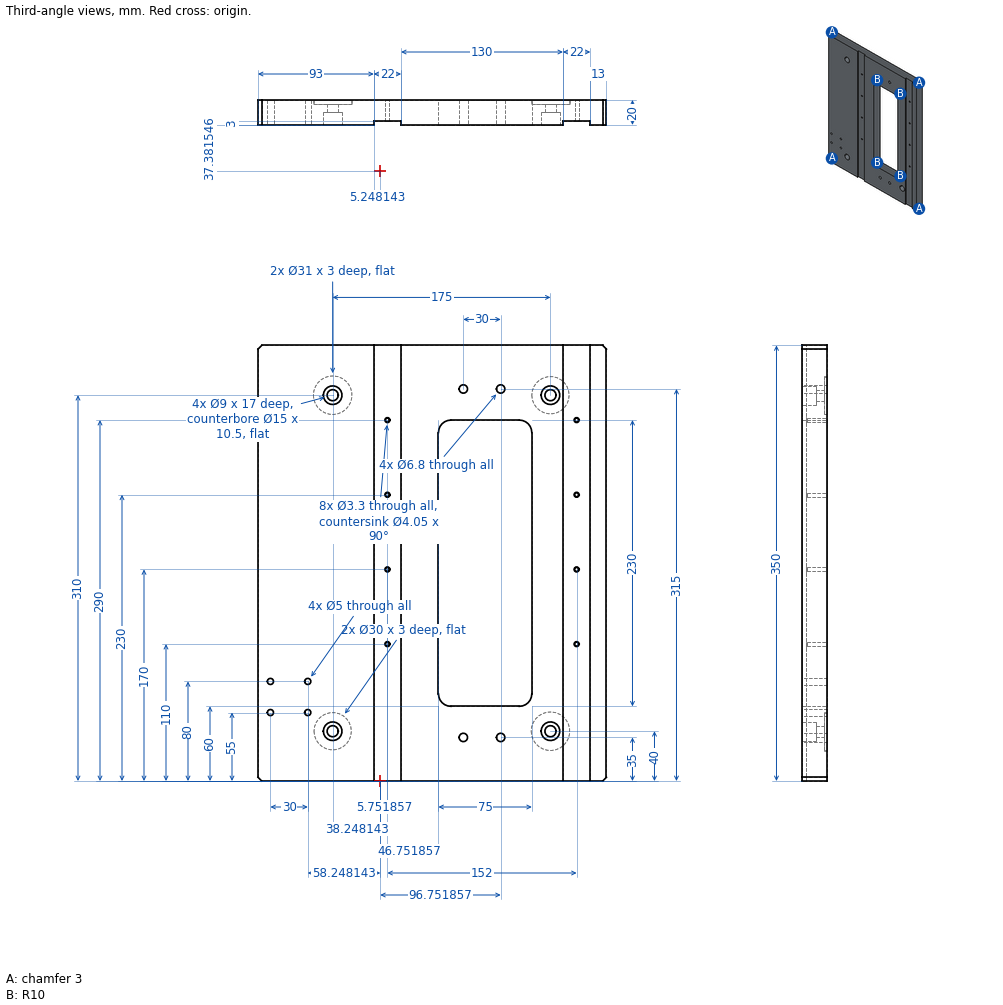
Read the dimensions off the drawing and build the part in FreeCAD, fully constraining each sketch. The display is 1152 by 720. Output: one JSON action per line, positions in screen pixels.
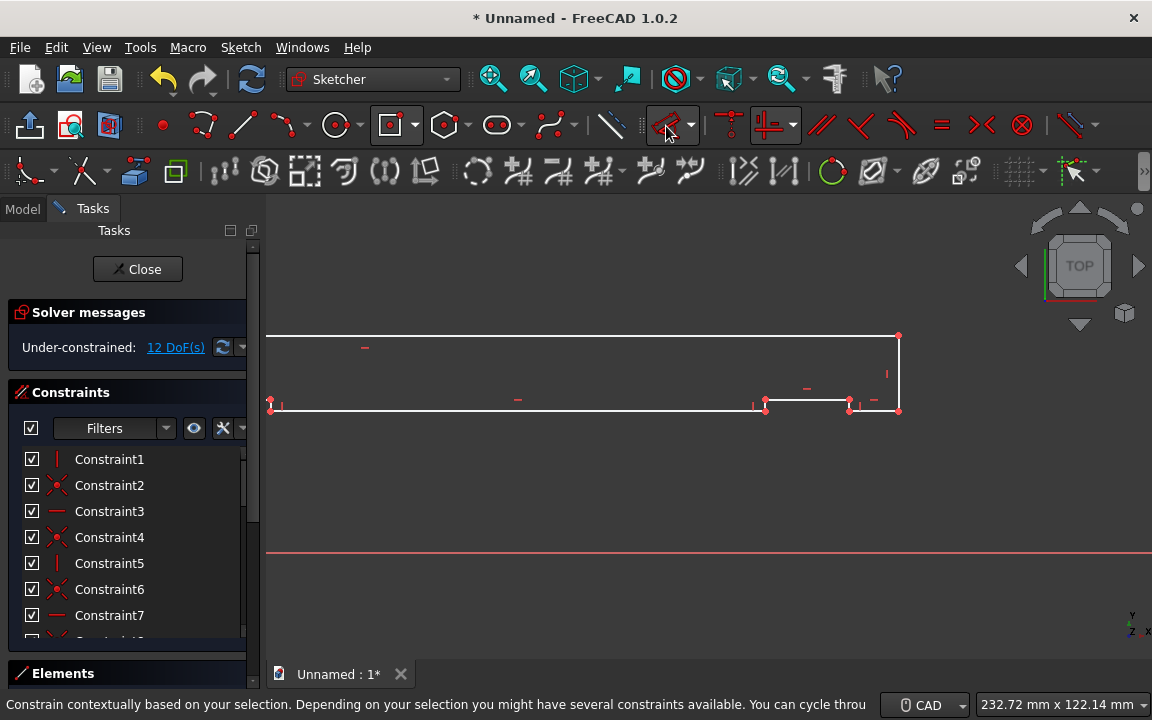
{"action": "scroll", "coordinate": [864, 412], "scroll_direction": "down", "scroll_amount": 4}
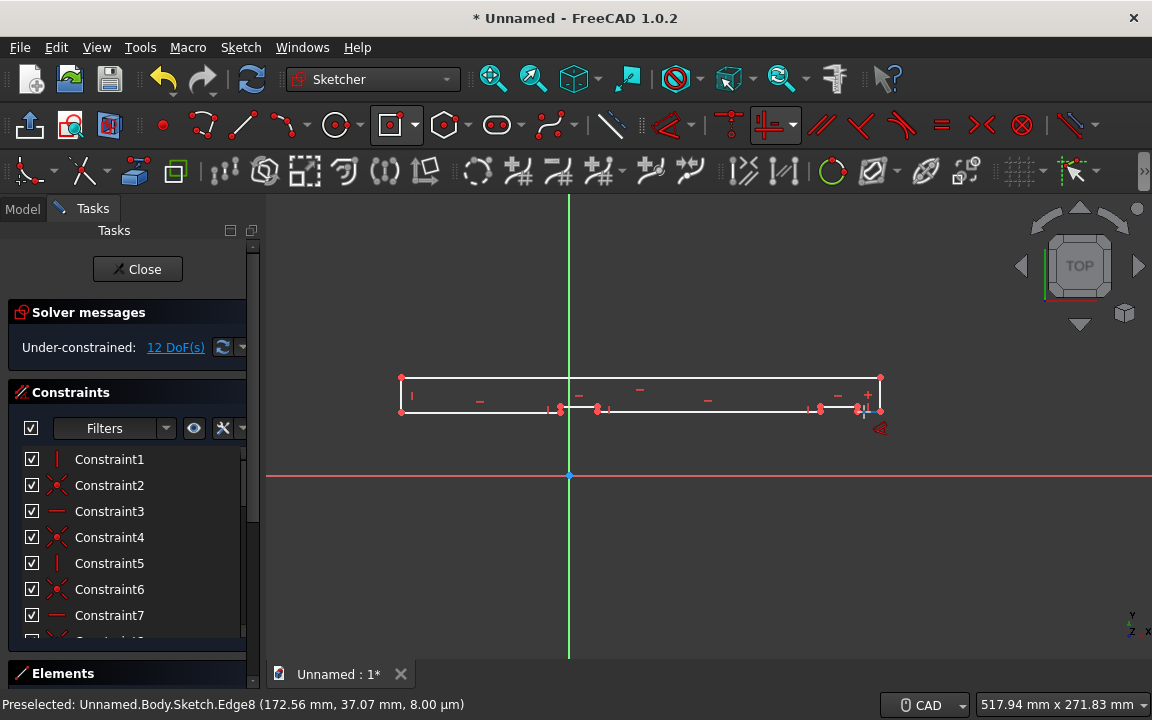
{"action": "scroll", "coordinate": [560, 410], "scroll_direction": "up", "scroll_amount": 11}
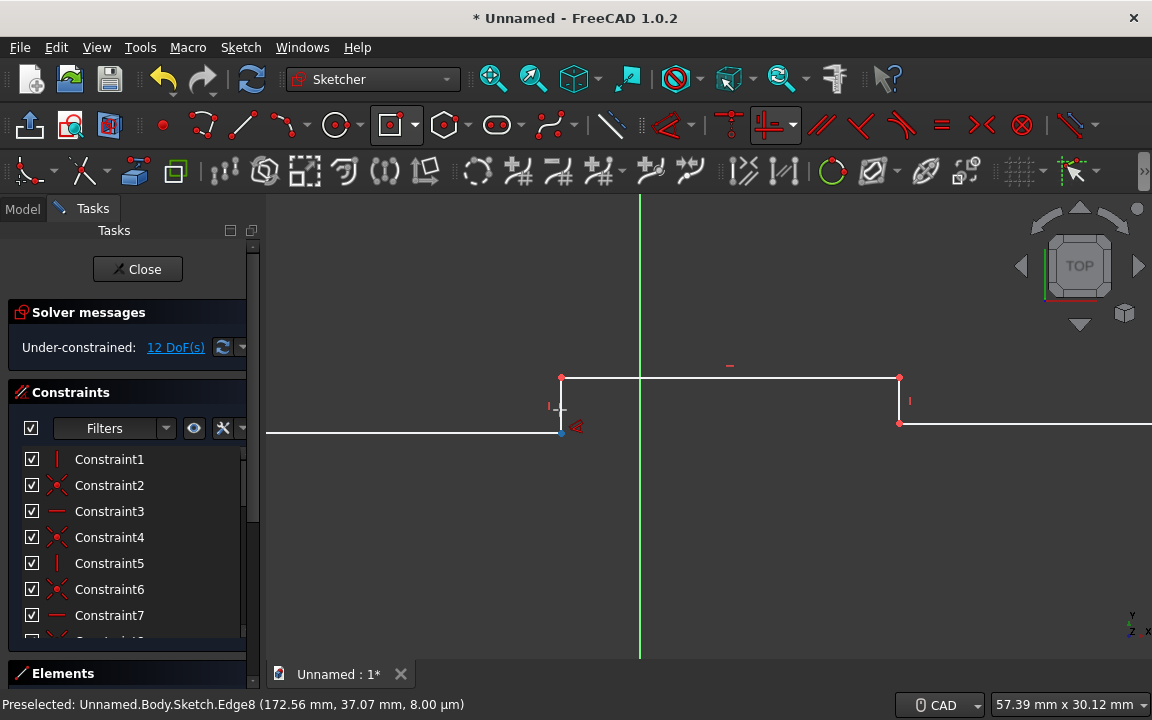
{"action": "left_click", "coordinate": [561, 405]}
{"action": "left_click", "coordinate": [527, 405]}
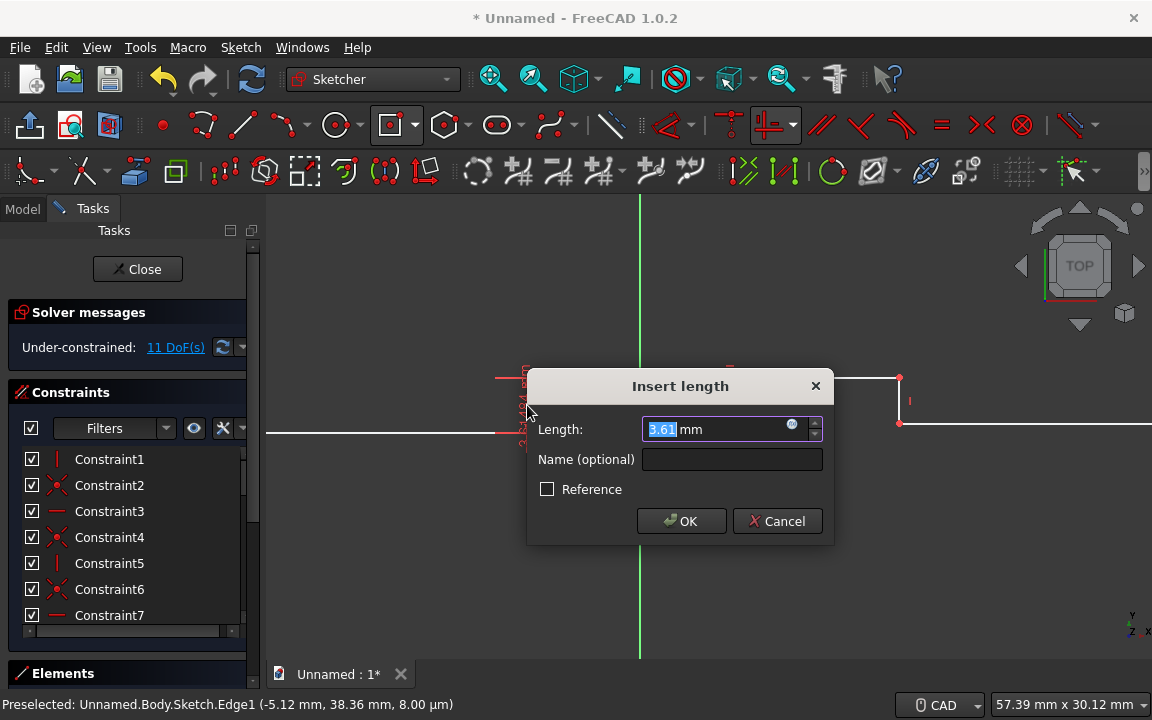
{"action": "type", "text": "3"}
{"action": "key", "text": "Return"}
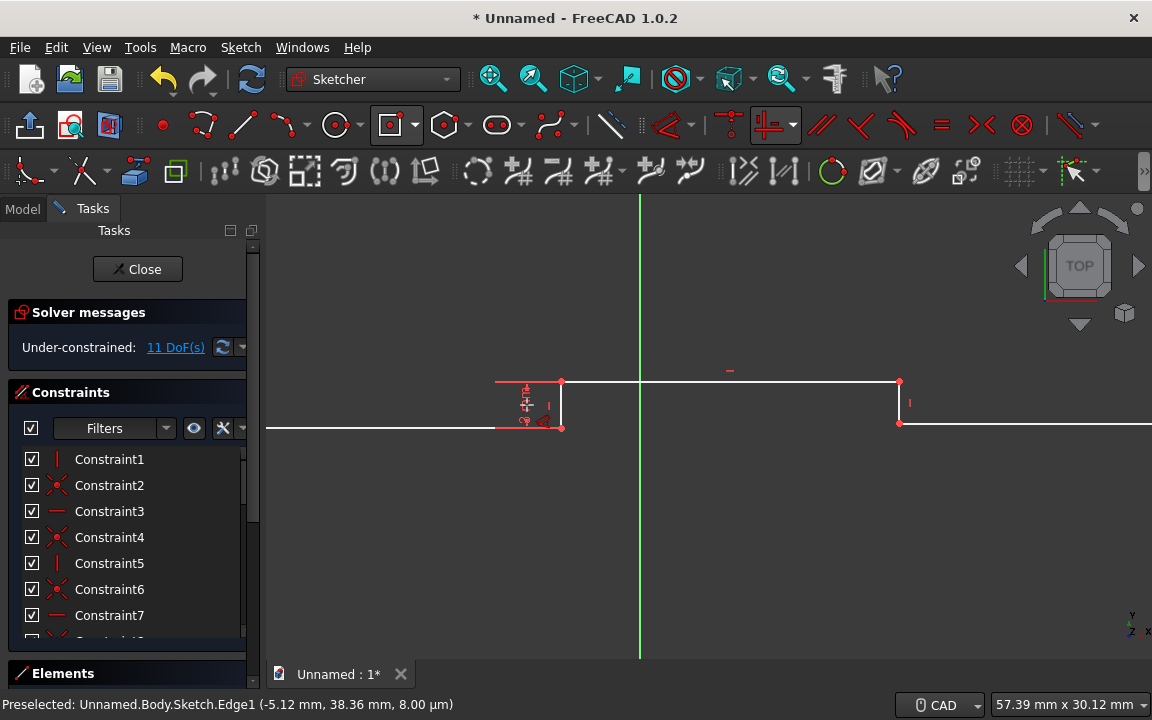
{"action": "left_click", "coordinate": [899, 394]}
{"action": "left_click", "coordinate": [865, 403]}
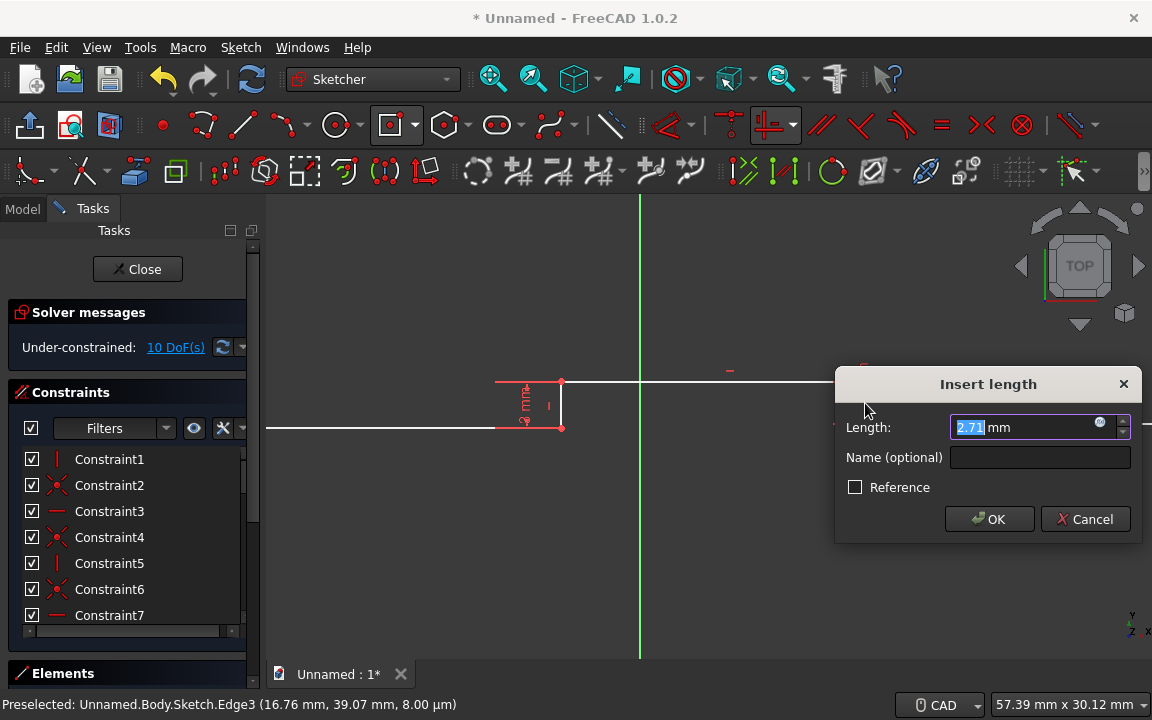
{"action": "type", "text": "3"}
{"action": "key", "text": "Return"}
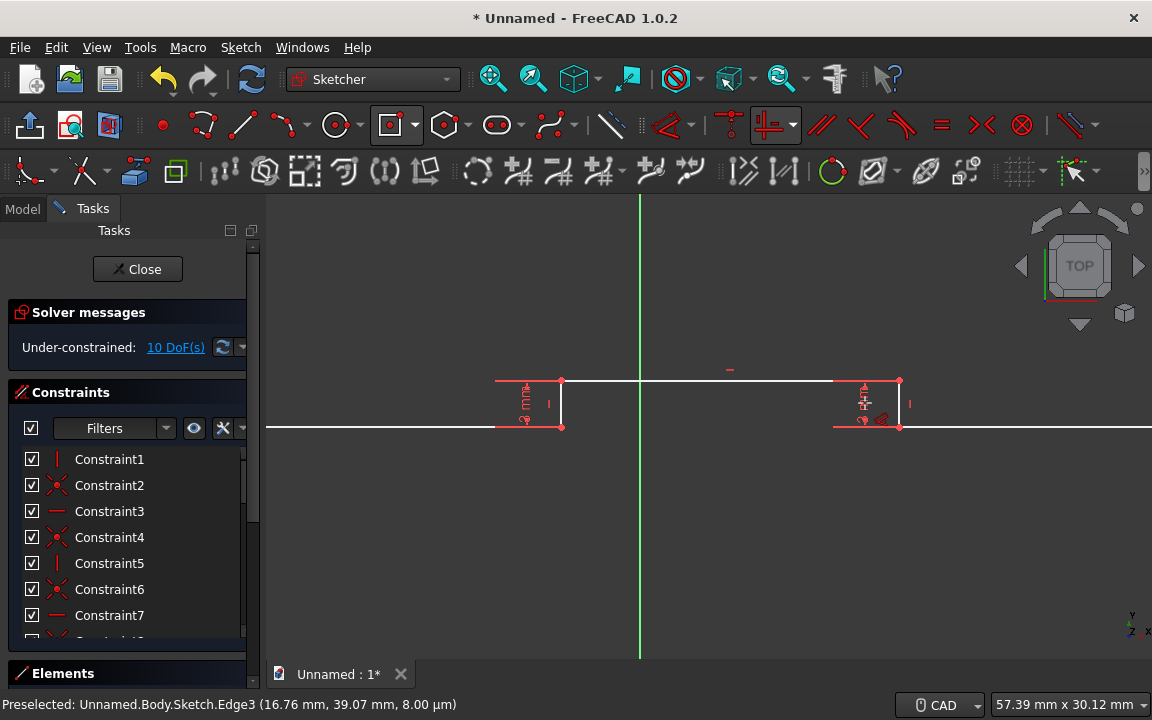
{"action": "scroll", "coordinate": [560, 410], "scroll_direction": "down", "scroll_amount": 11}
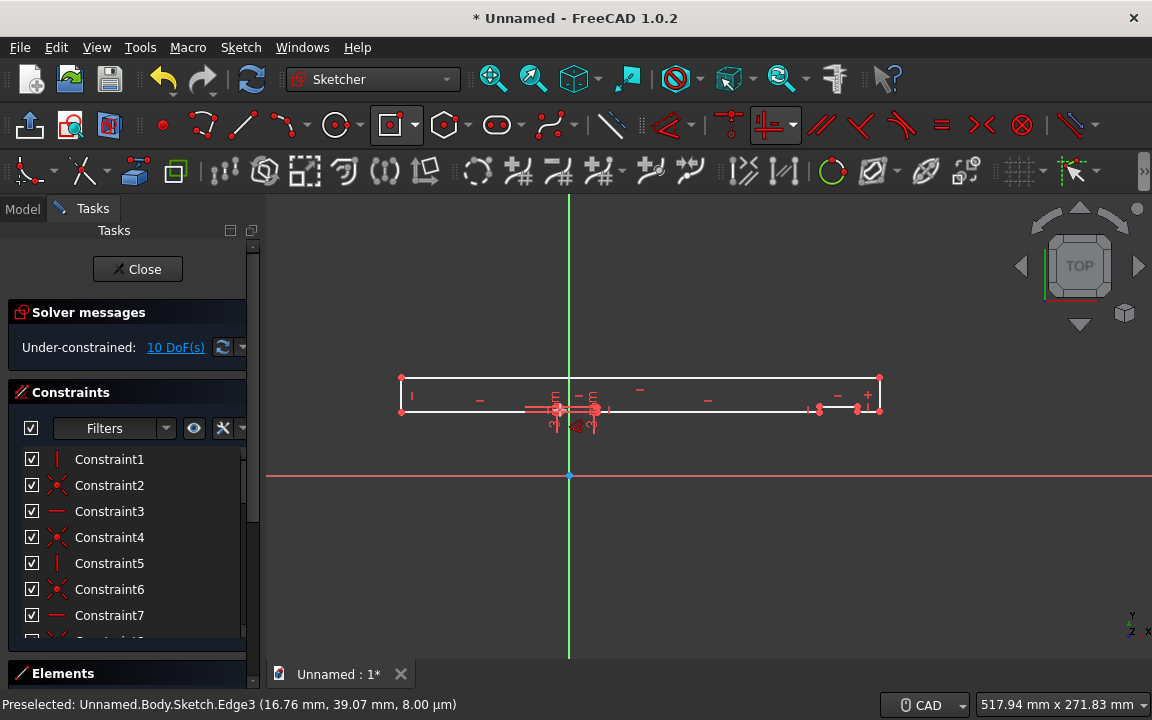
{"action": "scroll", "coordinate": [820, 411], "scroll_direction": "up", "scroll_amount": 11}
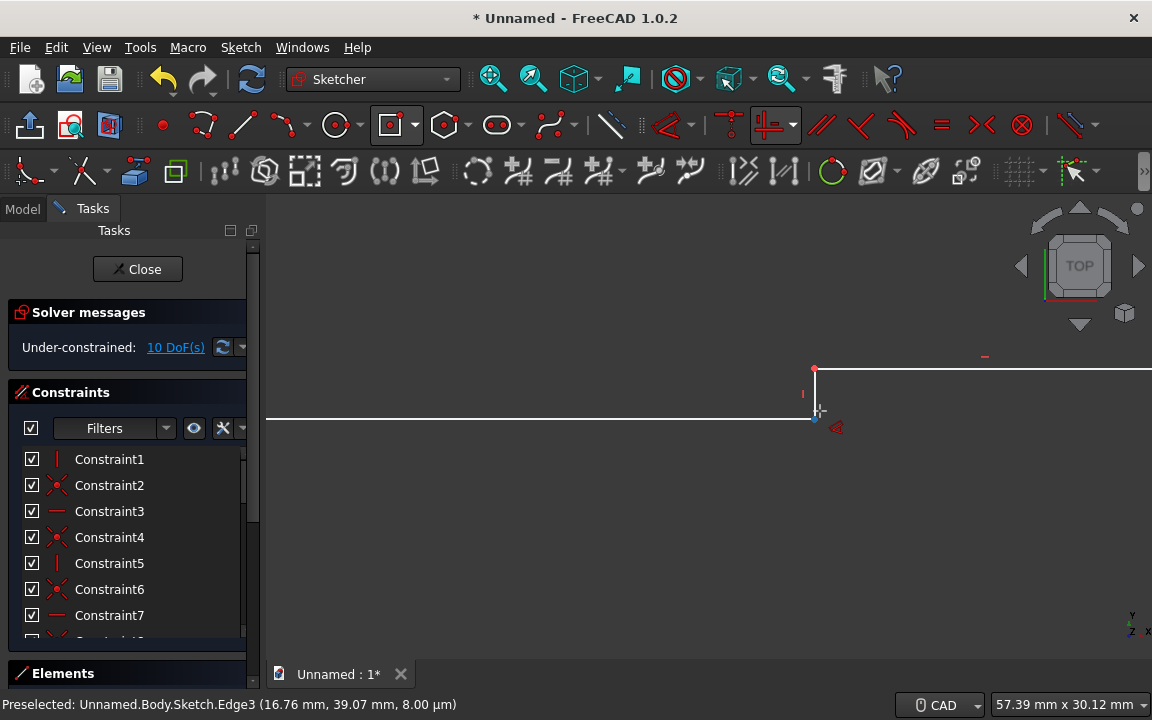
{"action": "left_click", "coordinate": [815, 404]}
{"action": "left_click", "coordinate": [849, 394]}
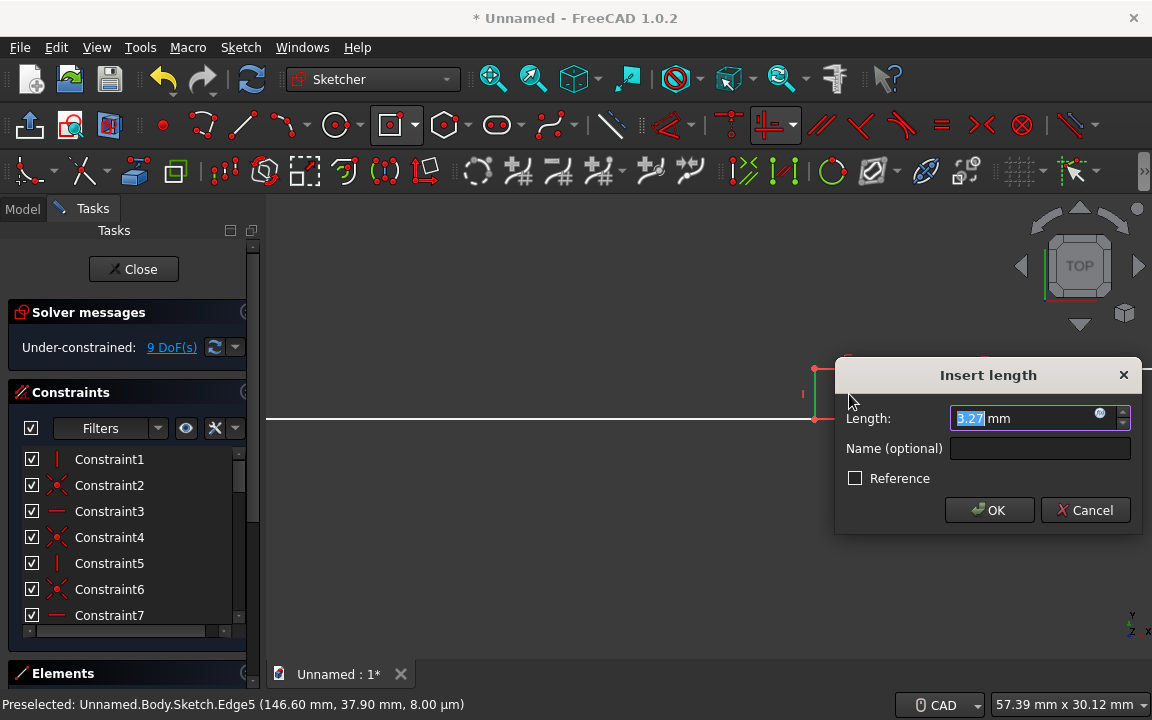
{"action": "type", "text": "3"}
{"action": "key", "text": "Return"}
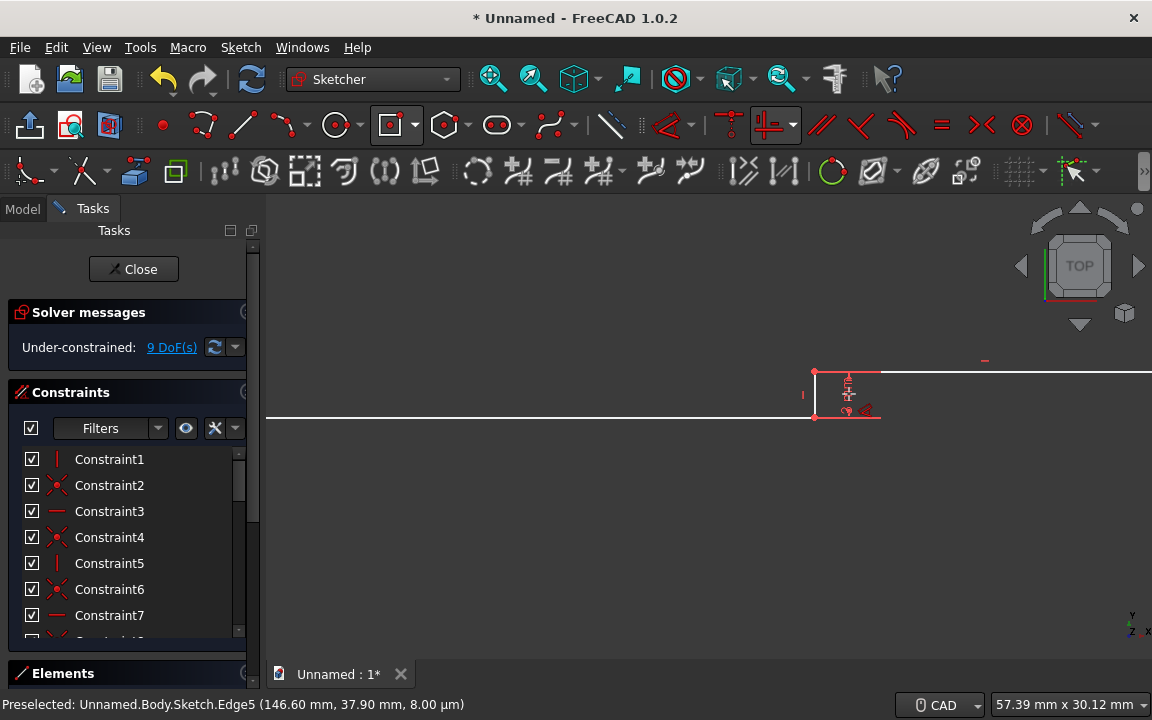
{"action": "scroll", "coordinate": [820, 411], "scroll_direction": "down", "scroll_amount": 11}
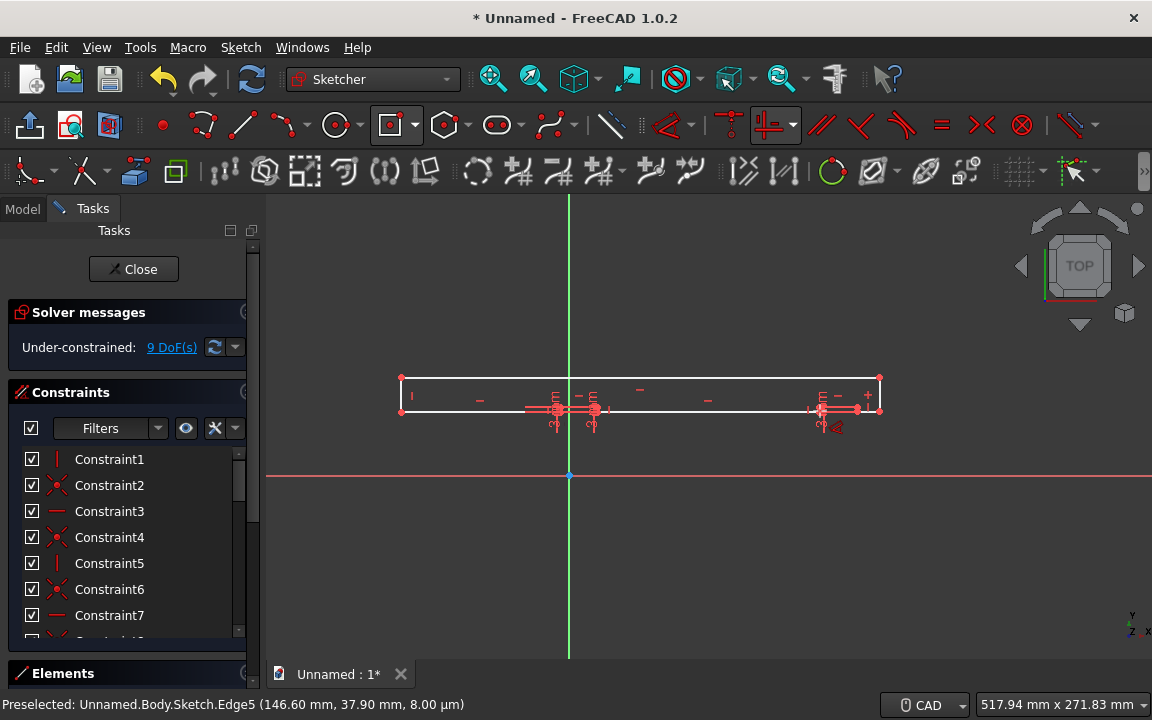
{"action": "scroll", "coordinate": [858, 408], "scroll_direction": "up", "scroll_amount": 12}